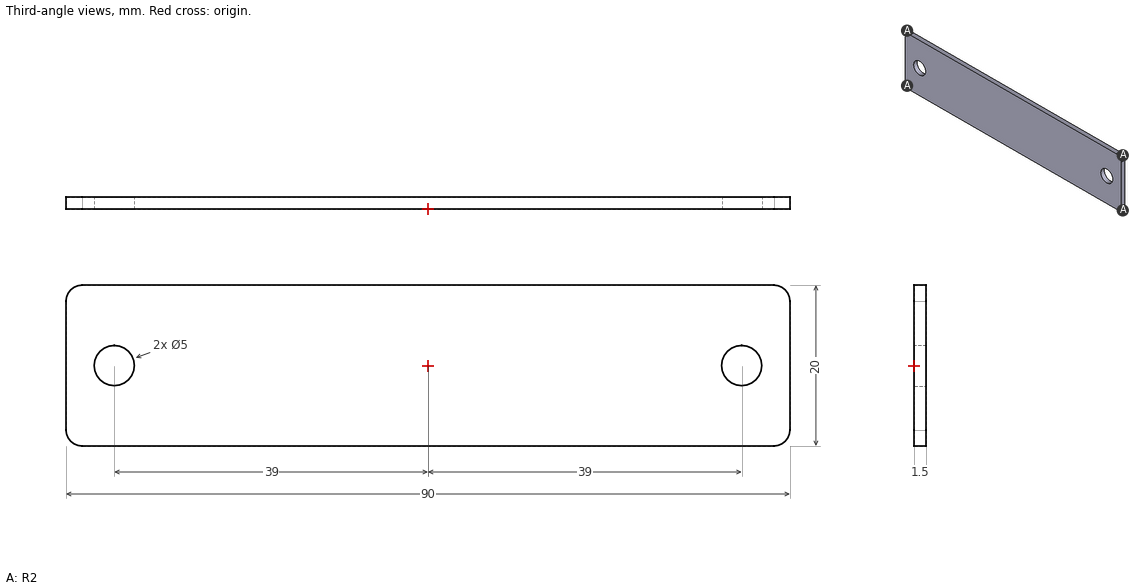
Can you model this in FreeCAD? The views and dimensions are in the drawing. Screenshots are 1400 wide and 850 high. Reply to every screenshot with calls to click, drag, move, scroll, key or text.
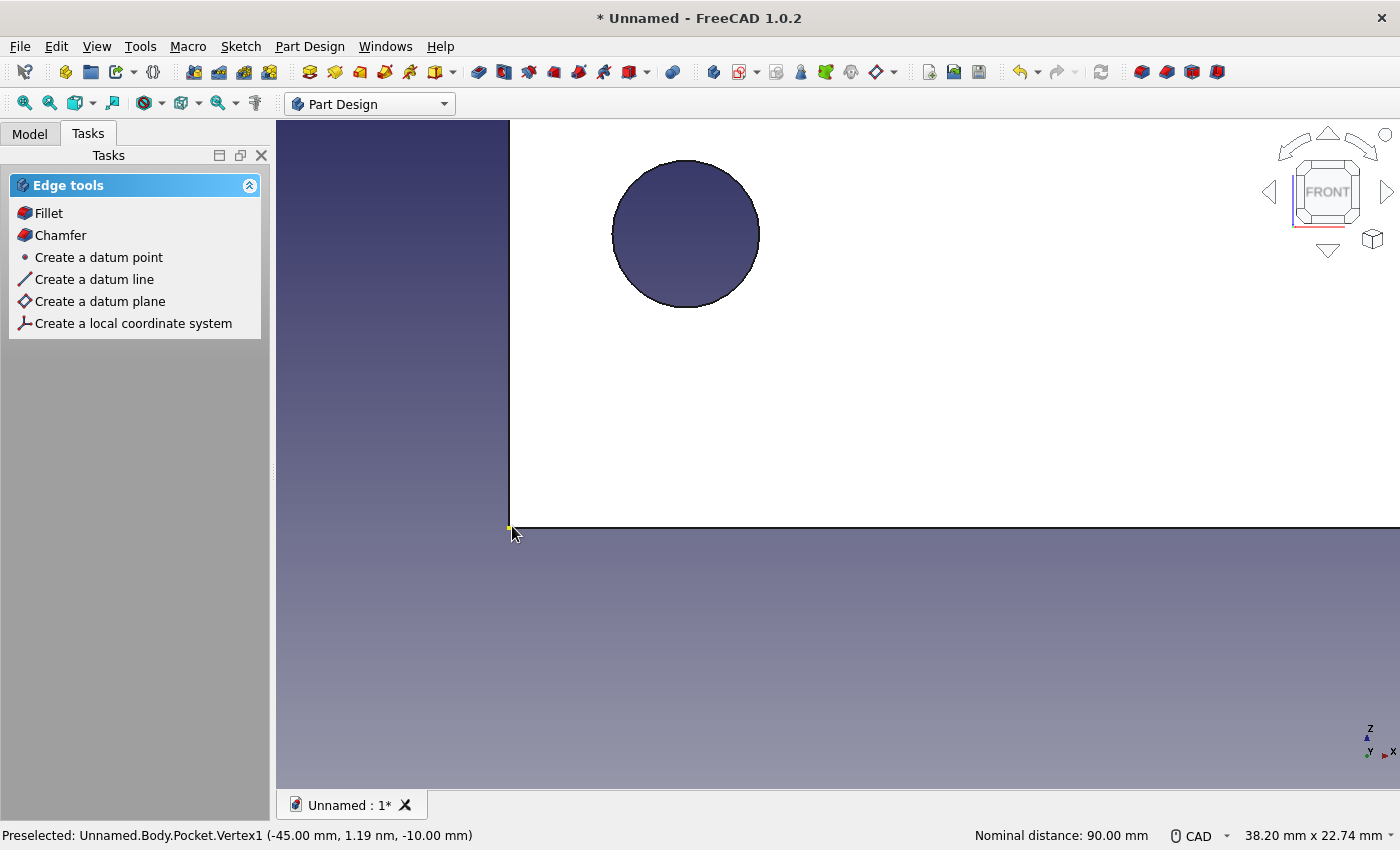
click(25, 104)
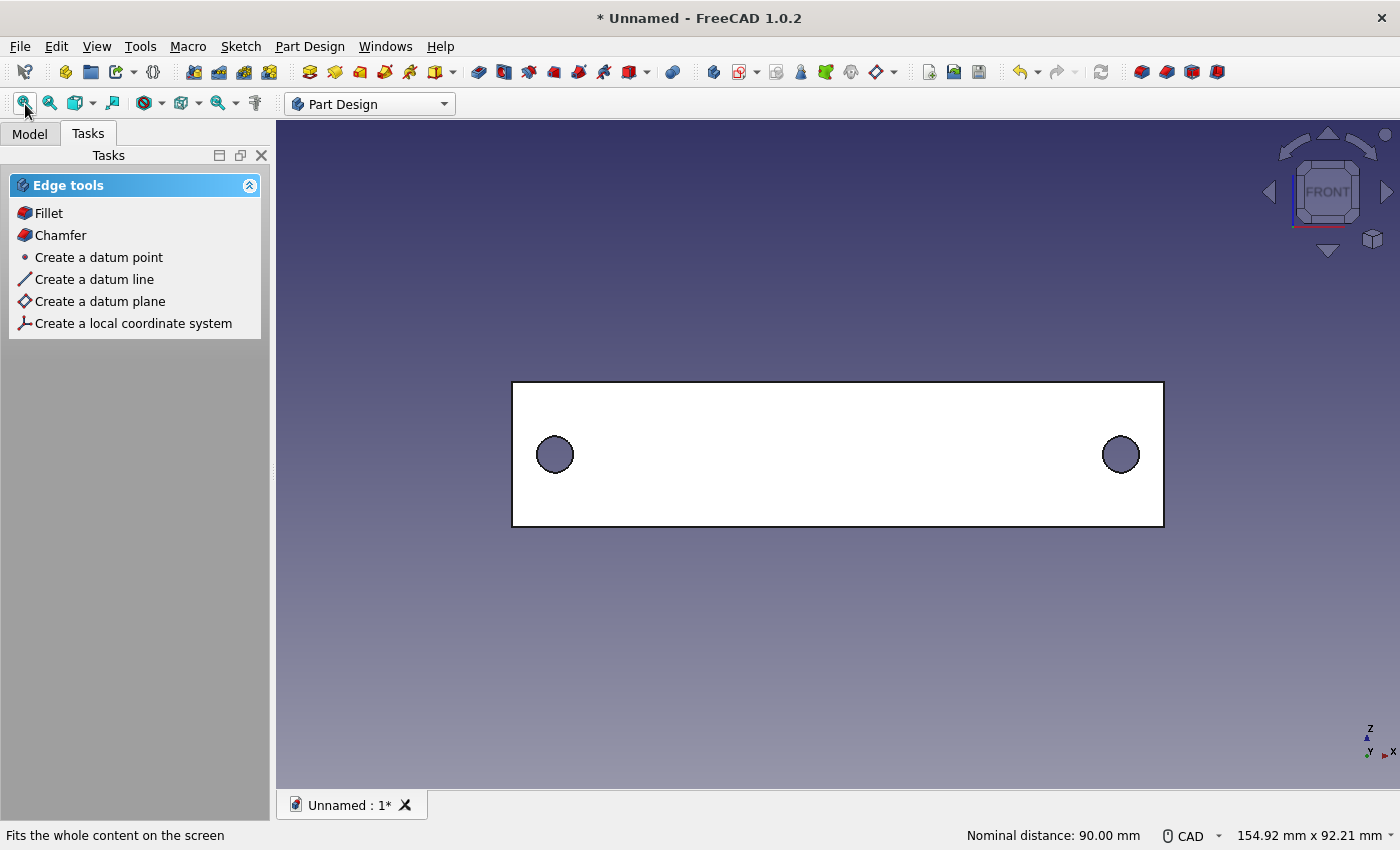
key(3)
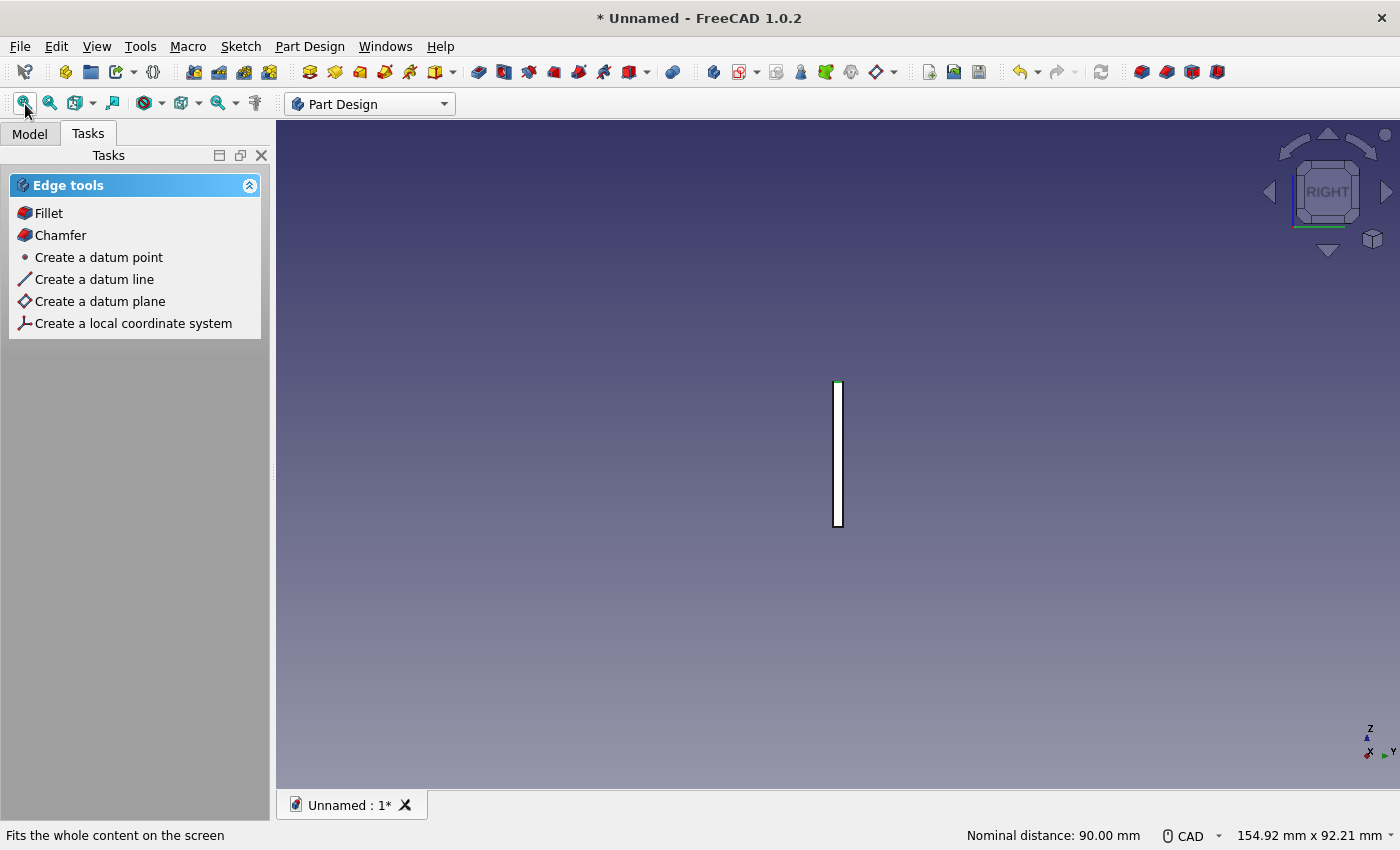
click(25, 104)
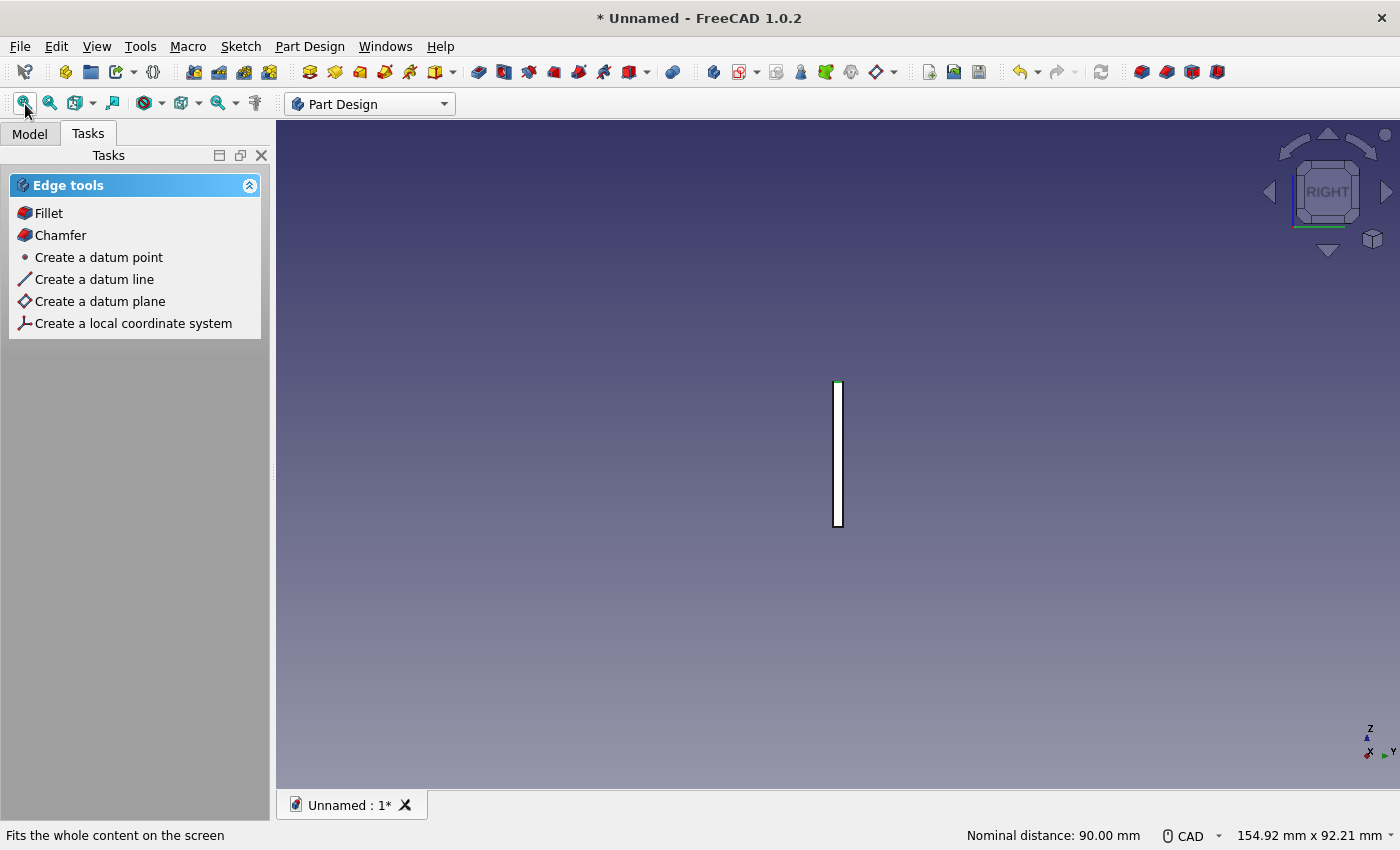
scroll(838, 526, up, 7)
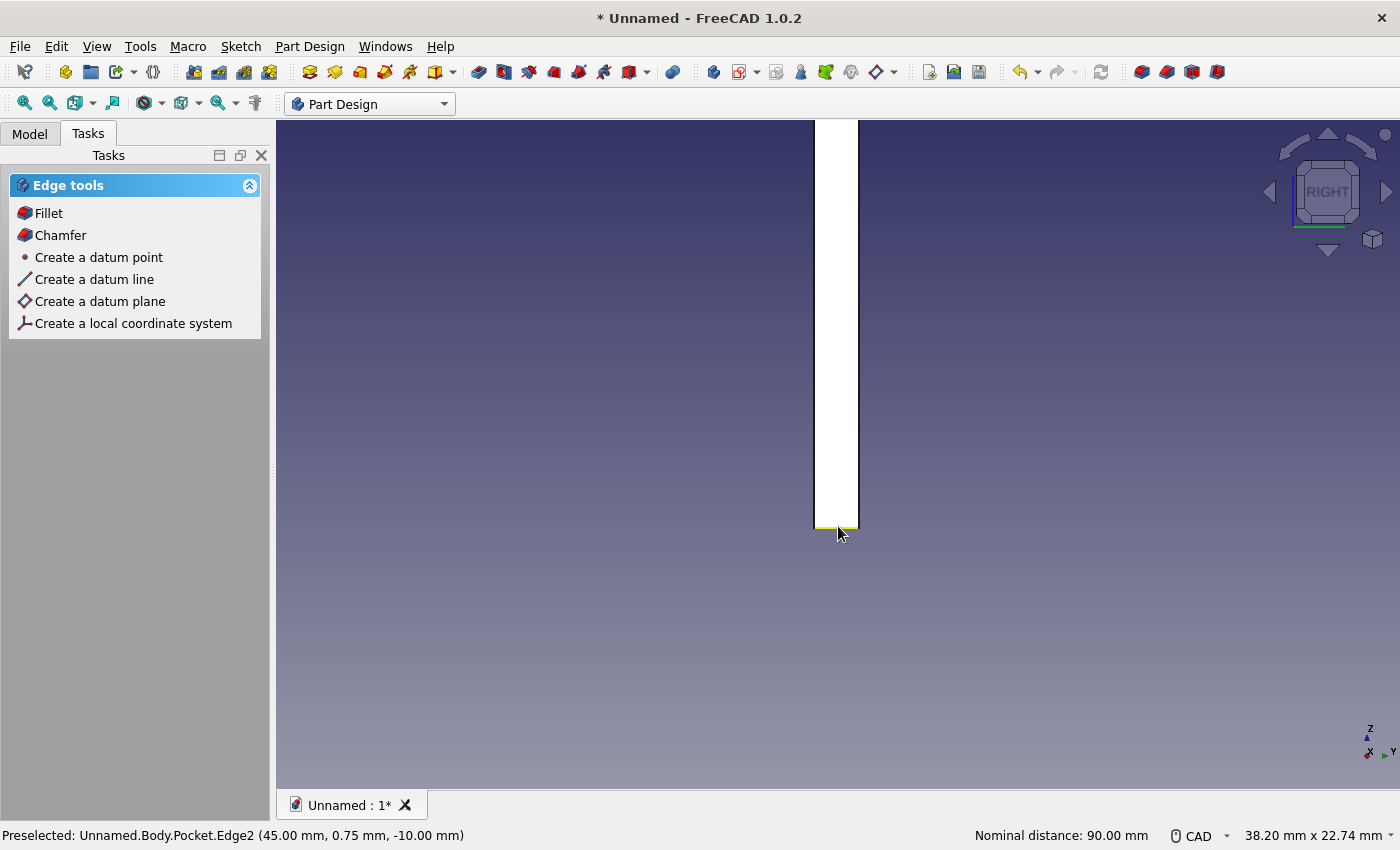
click(836, 527, ctrl)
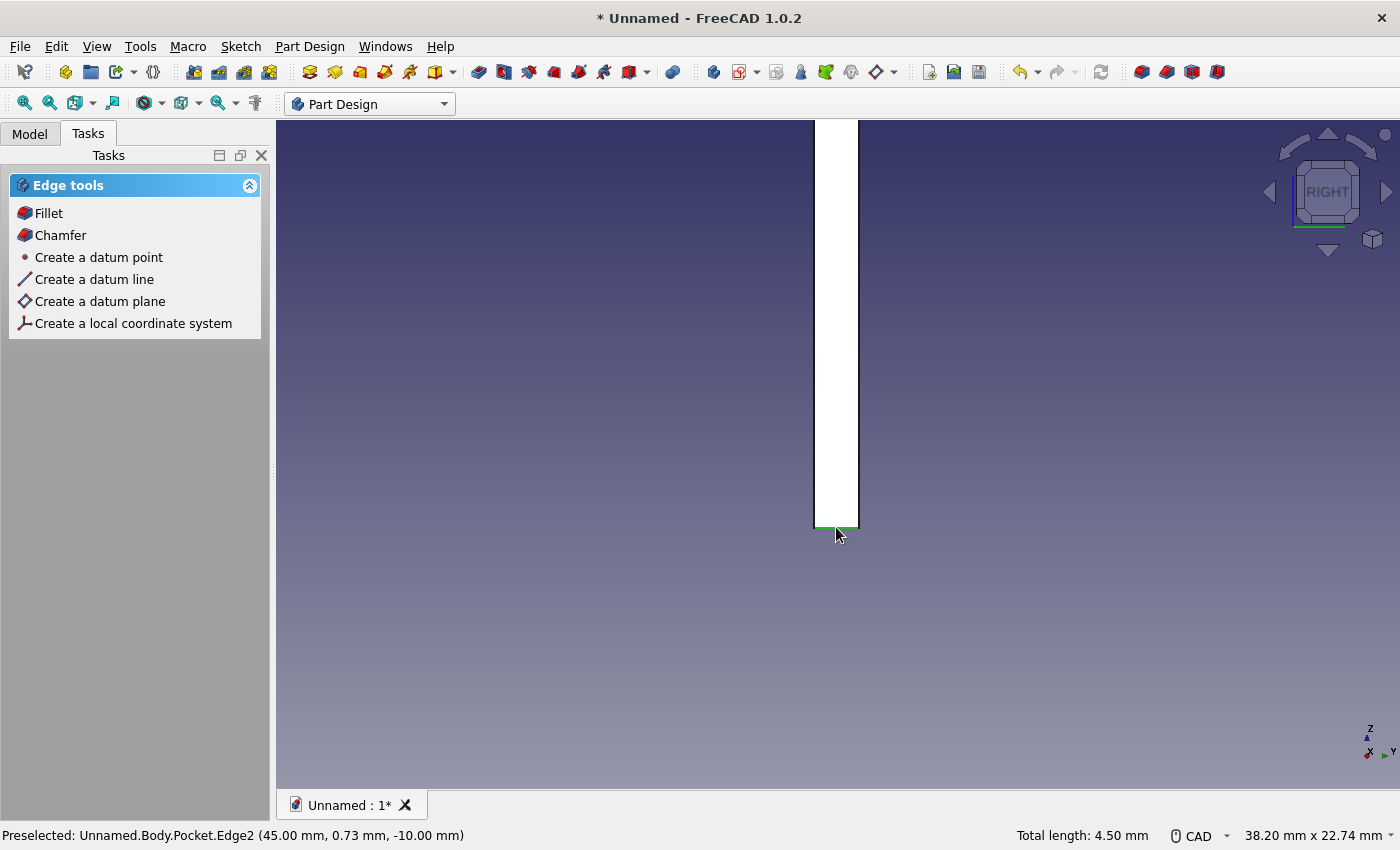
click(25, 104)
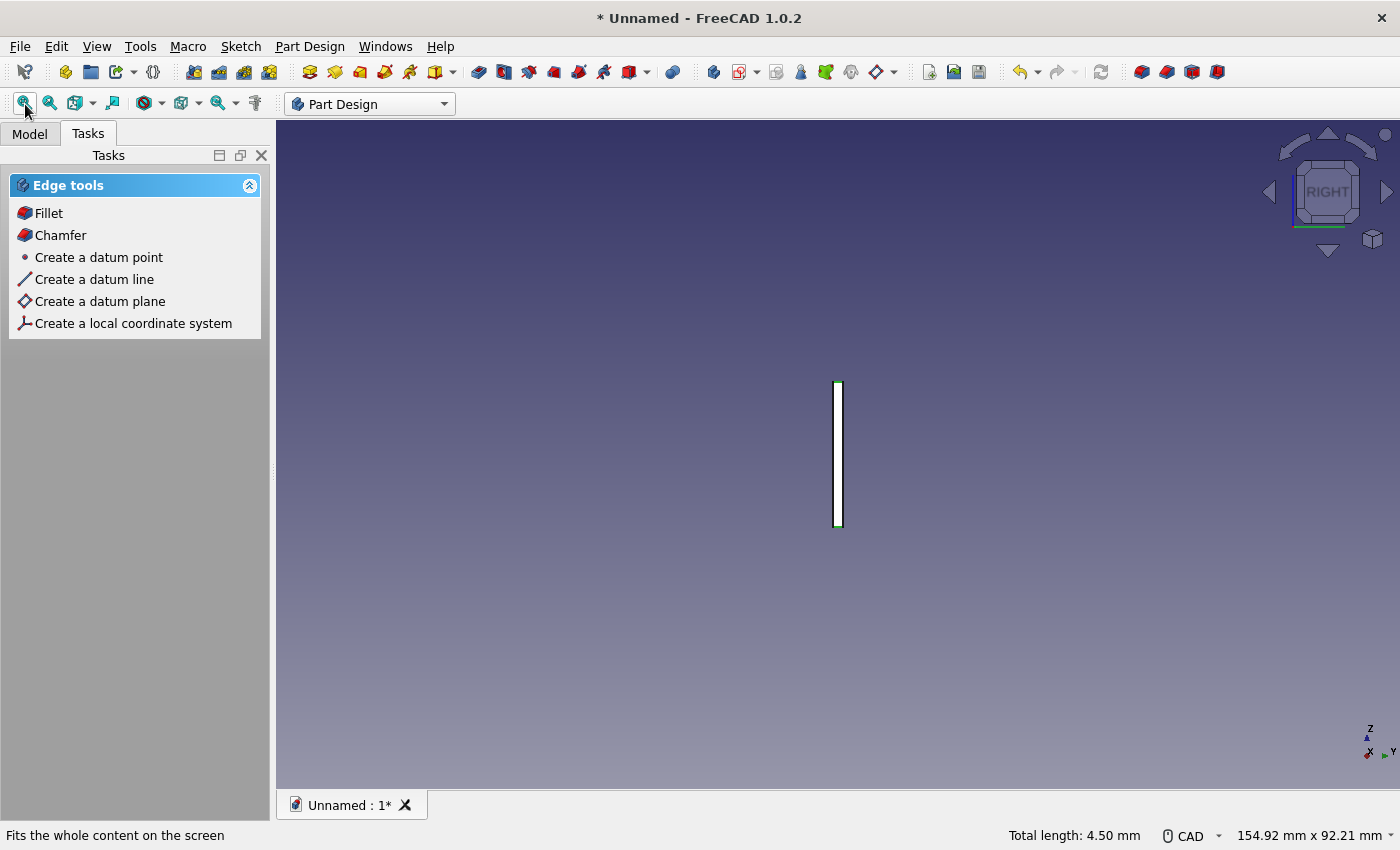
key(5)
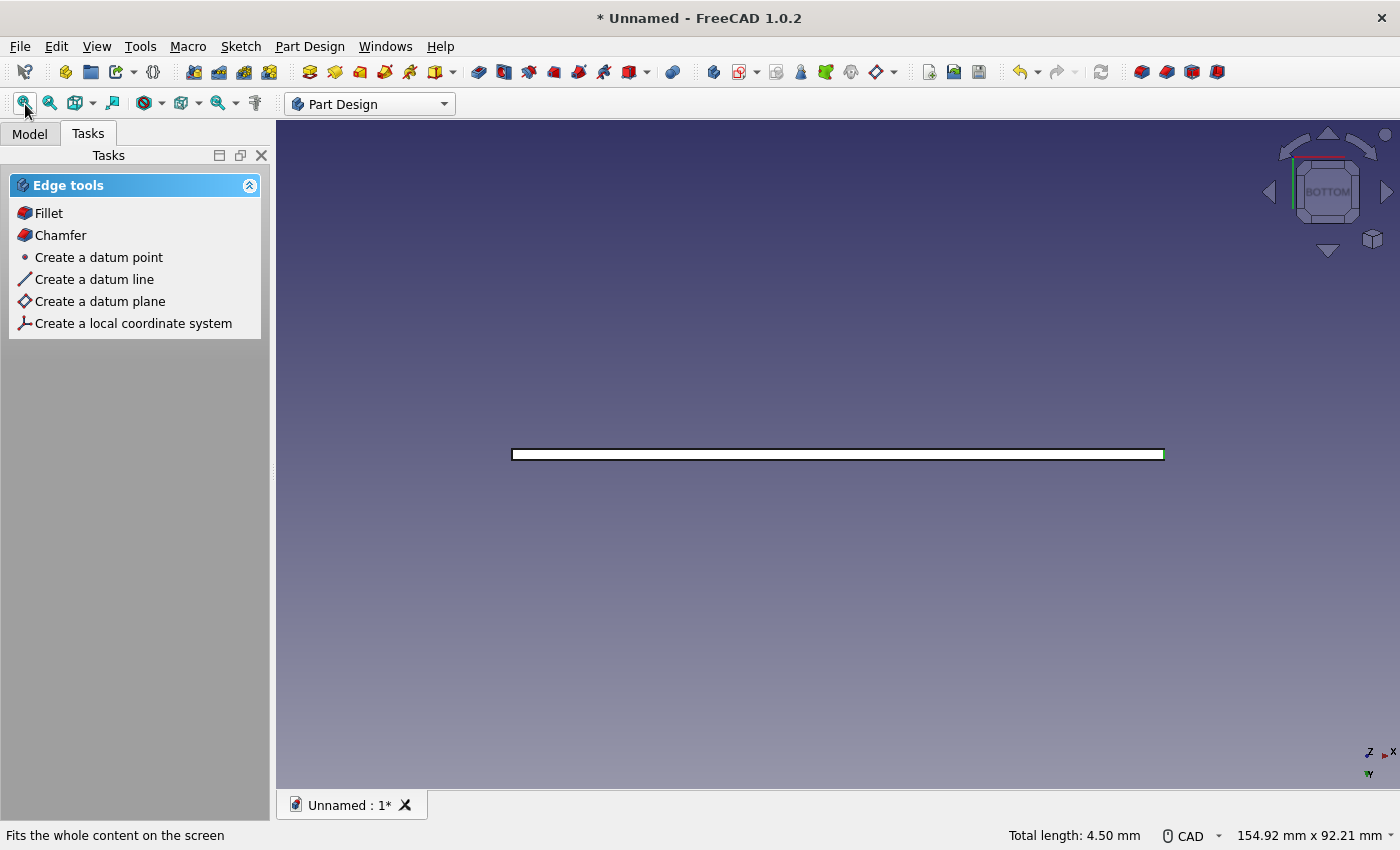
click(512, 455, ctrl)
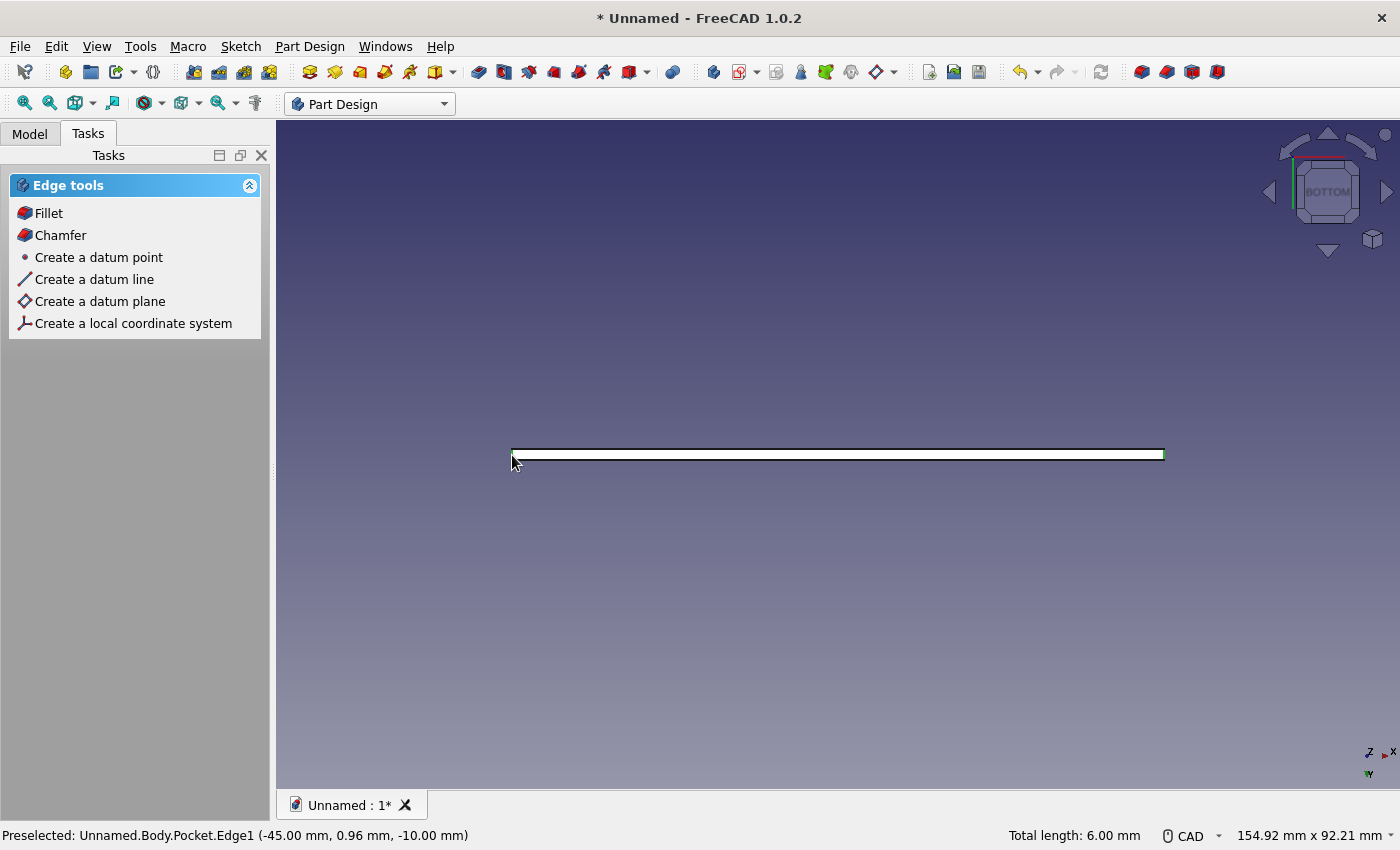
click(1142, 72)